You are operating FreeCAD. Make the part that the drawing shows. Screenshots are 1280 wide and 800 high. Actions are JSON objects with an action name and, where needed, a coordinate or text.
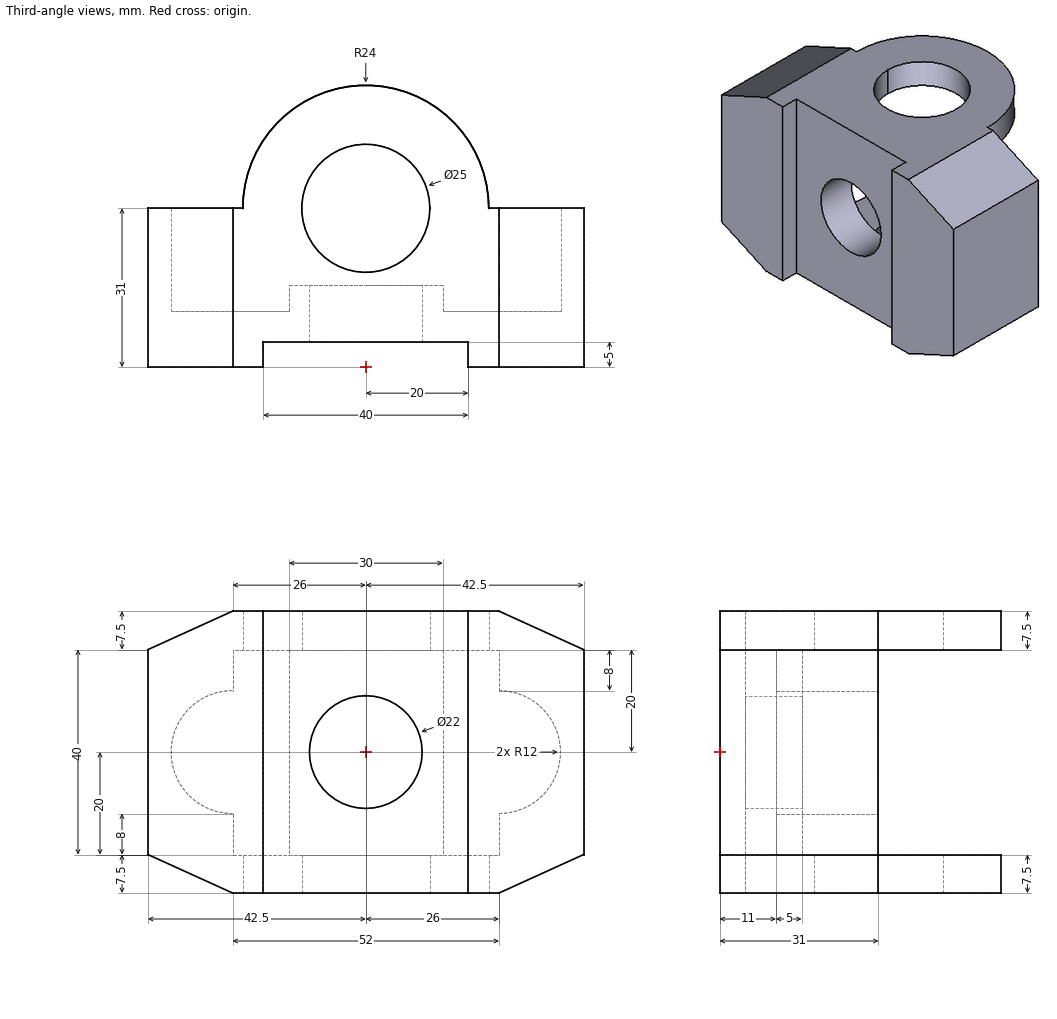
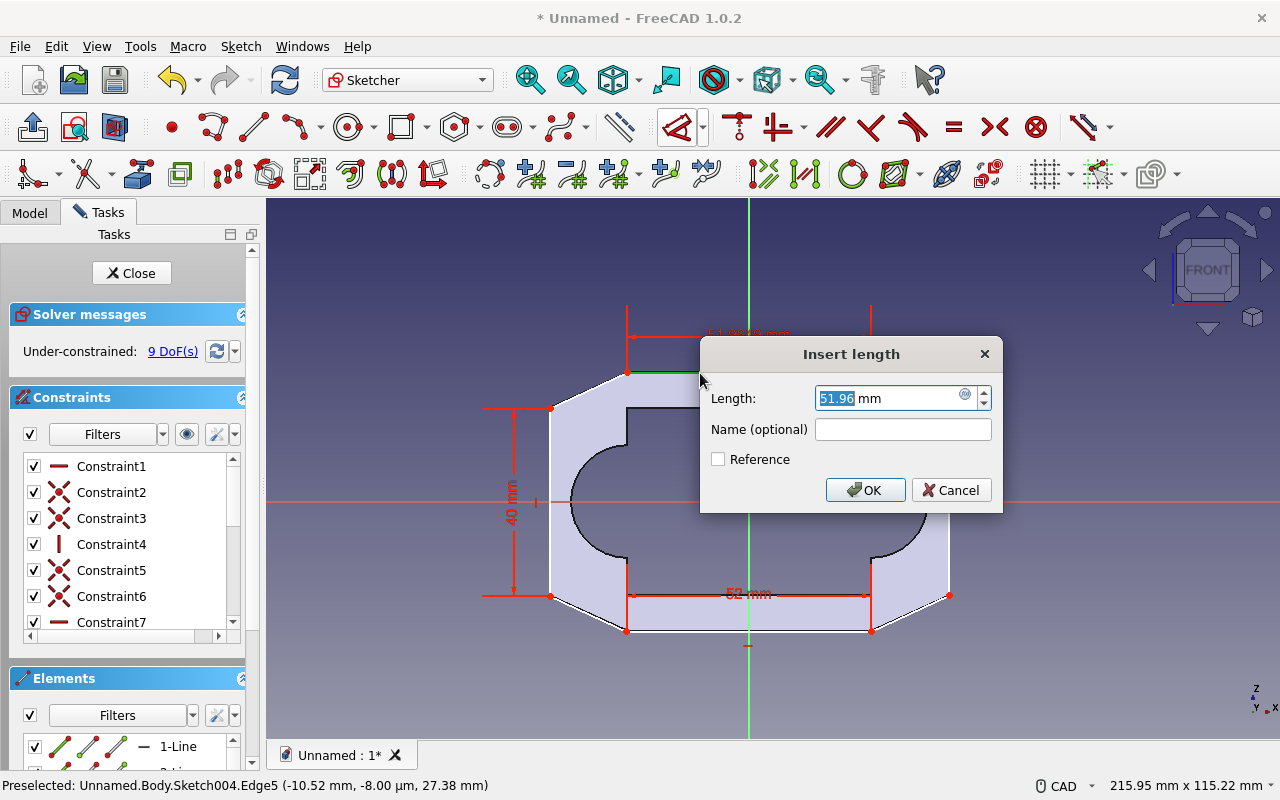
{"action": "type", "text": "52"}
{"action": "key", "text": "Return"}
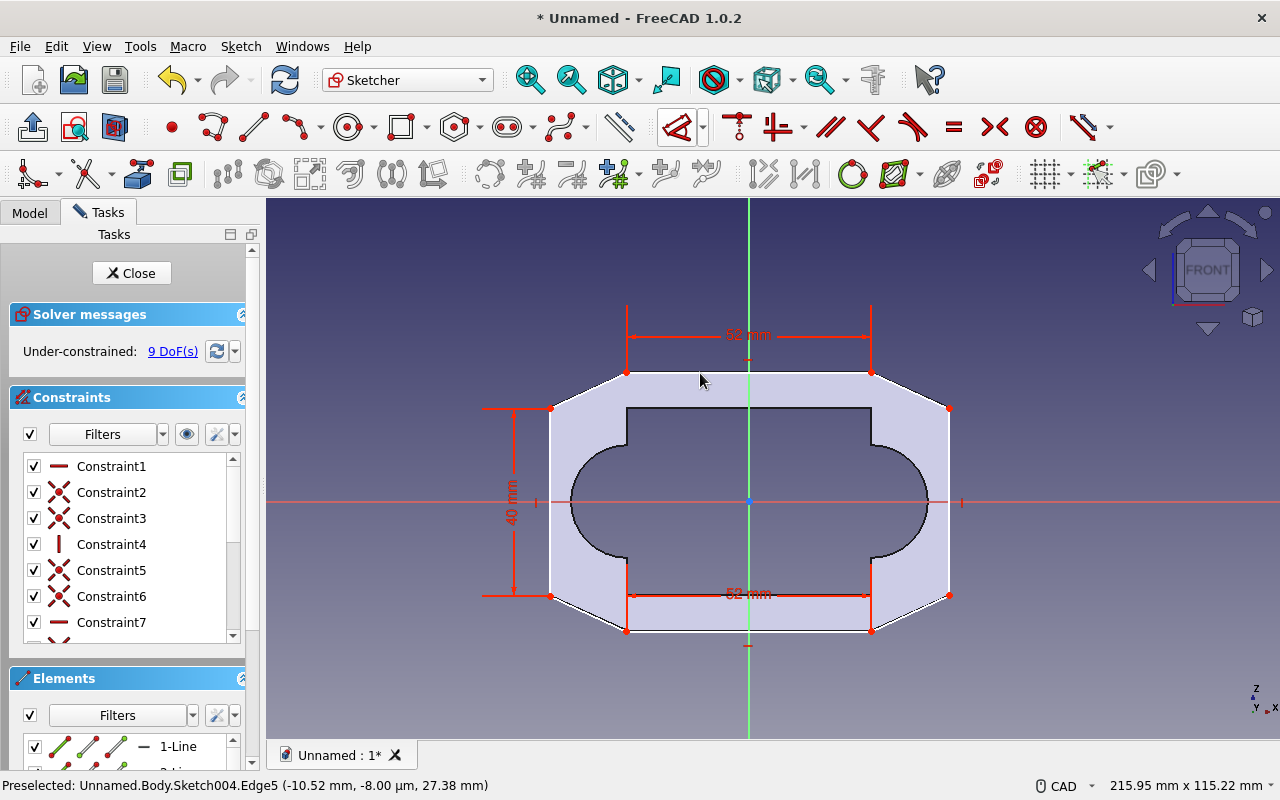
{"action": "left_click", "coordinate": [949, 465]}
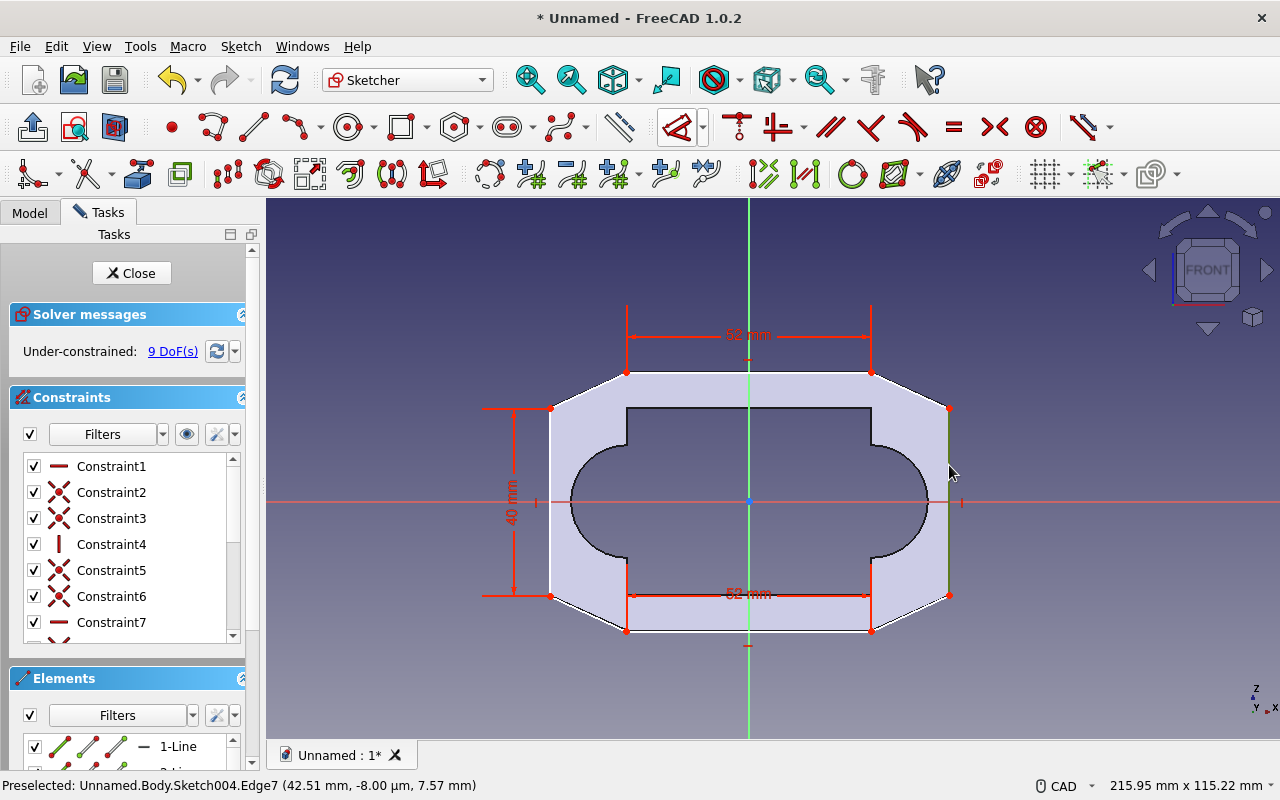
{"action": "key", "text": "i"}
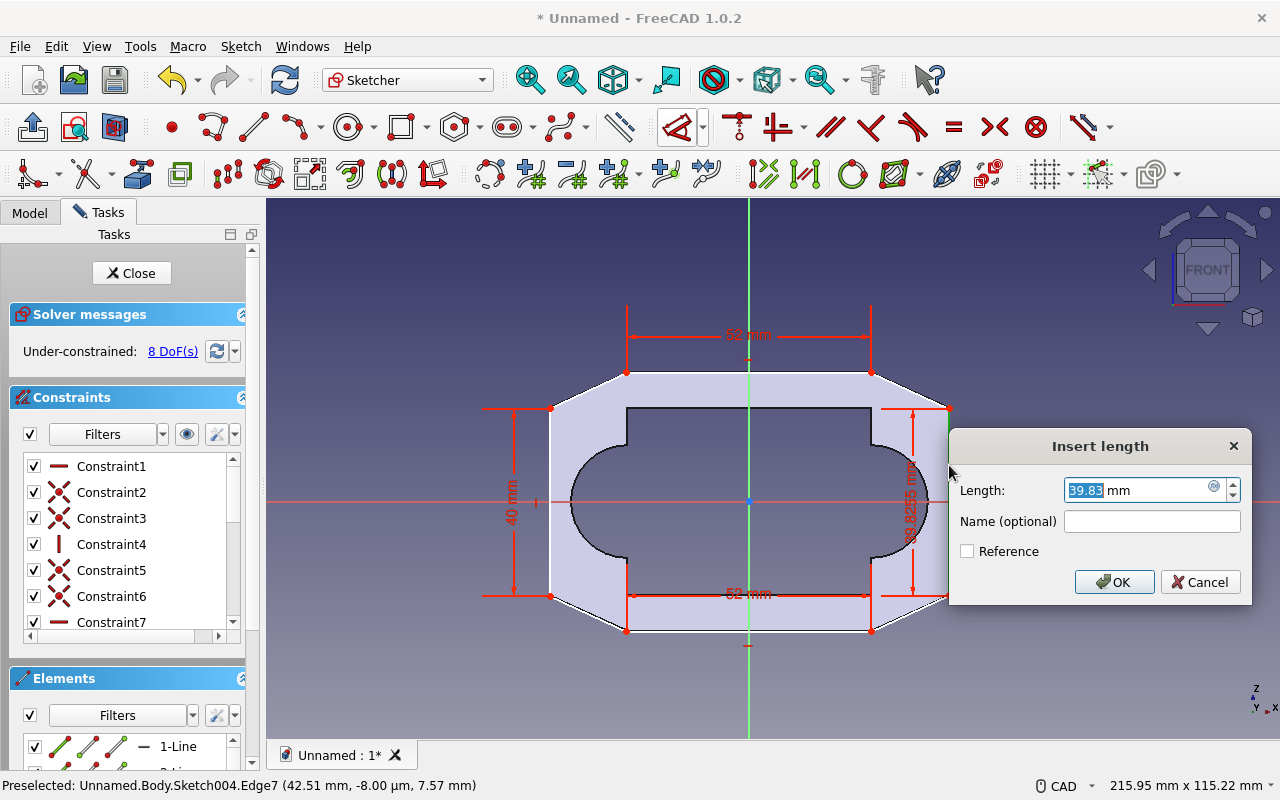
{"action": "type", "text": "40"}
{"action": "key", "text": "Return"}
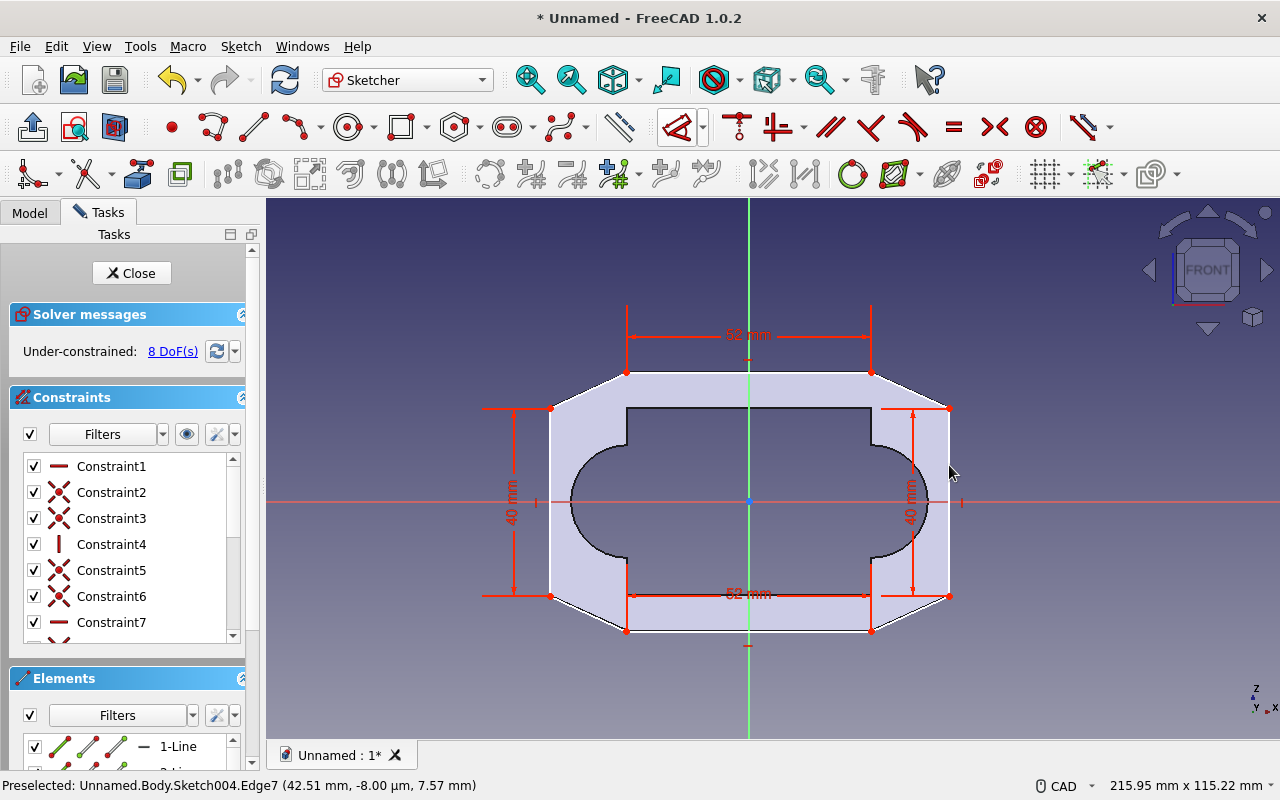
{"action": "left_click", "coordinate": [871, 632]}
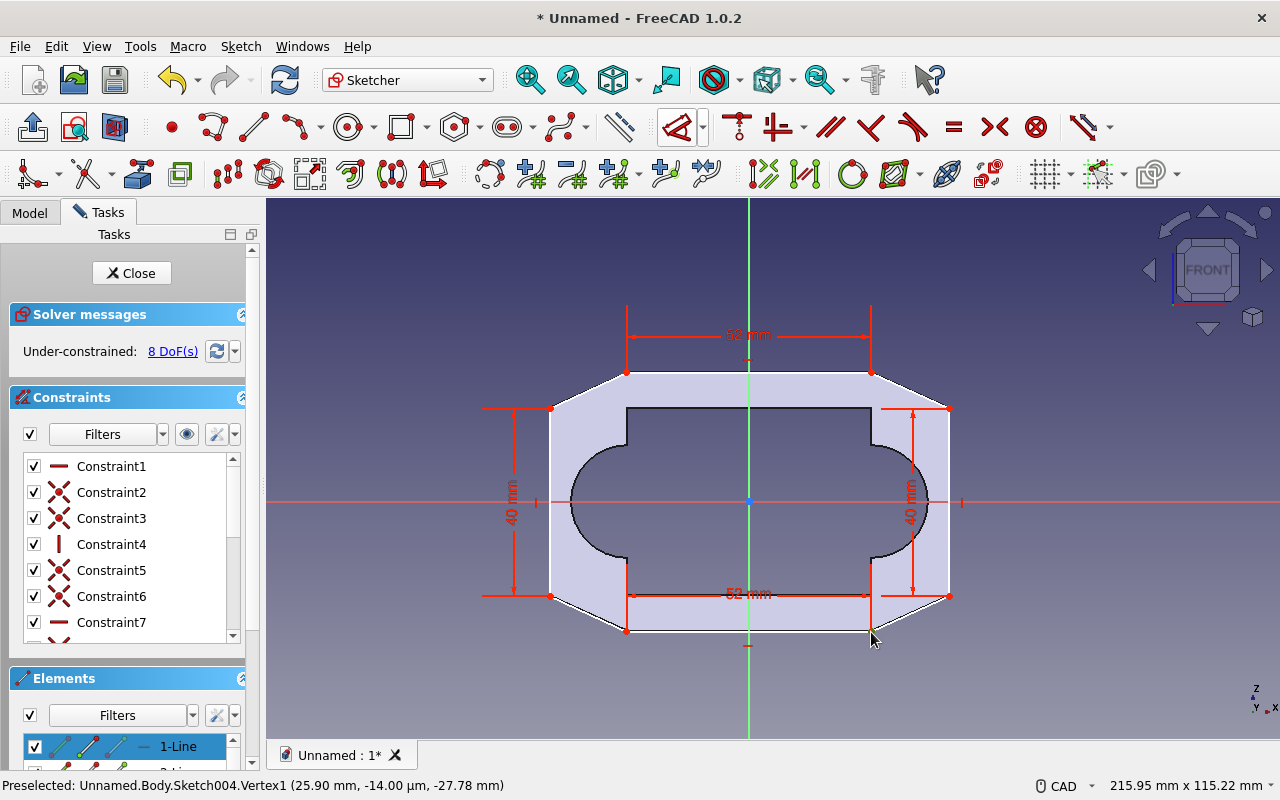
{"action": "key", "text": "l"}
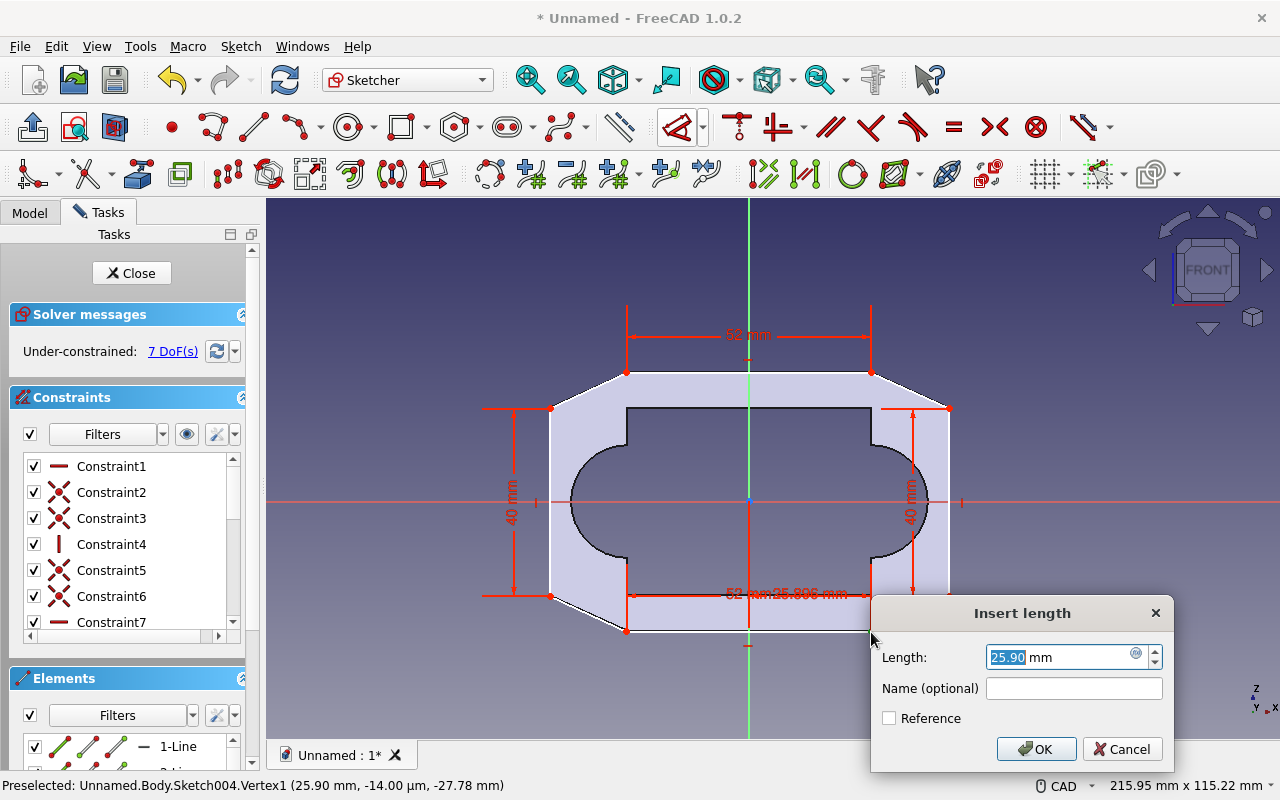
{"action": "type", "text": "26"}
{"action": "key", "text": "Return"}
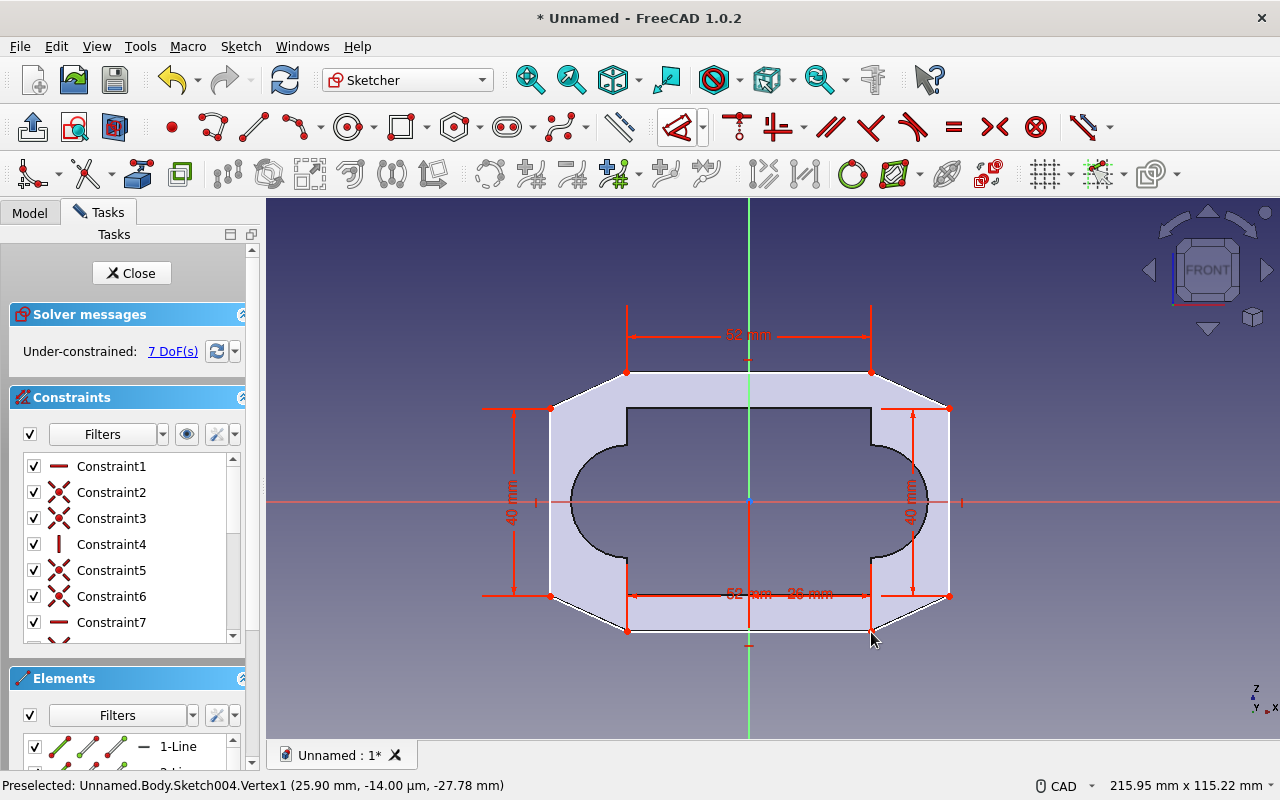
{"action": "left_click", "coordinate": [550, 596]}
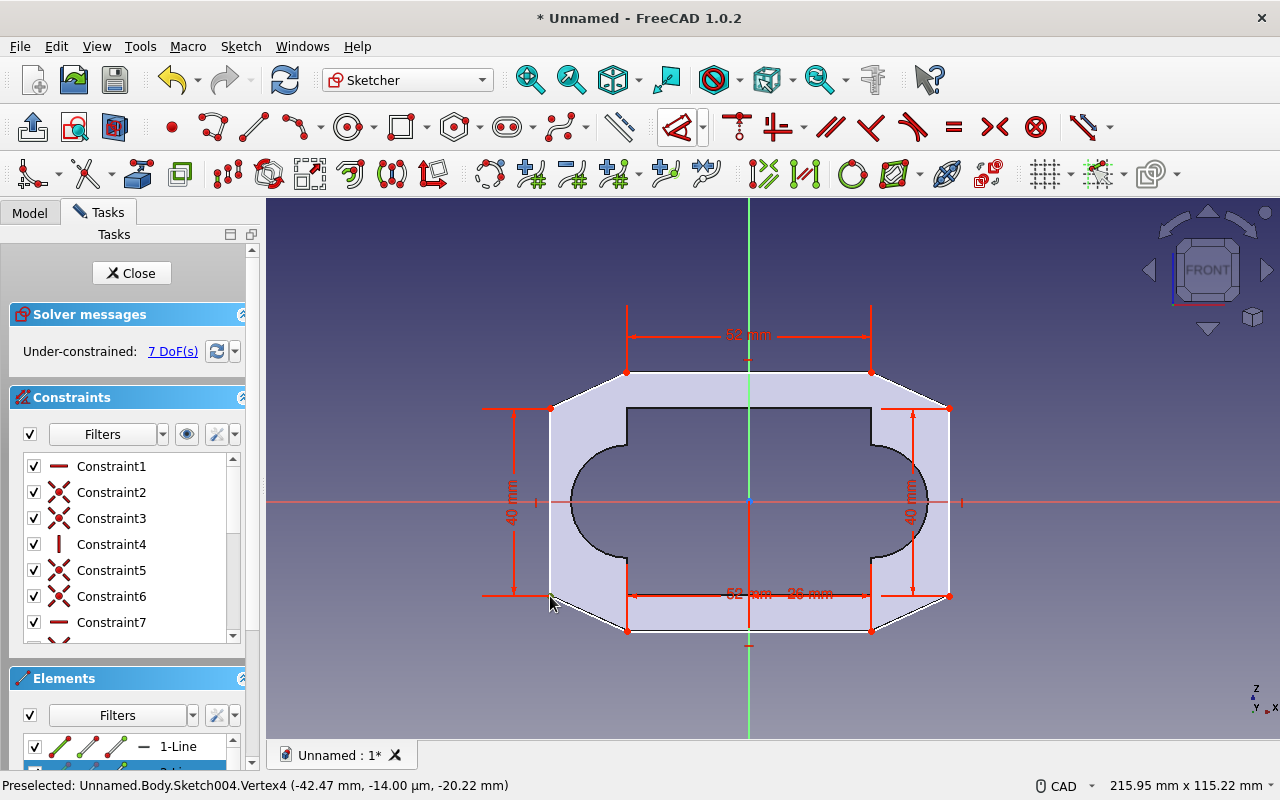
{"action": "key", "text": "i"}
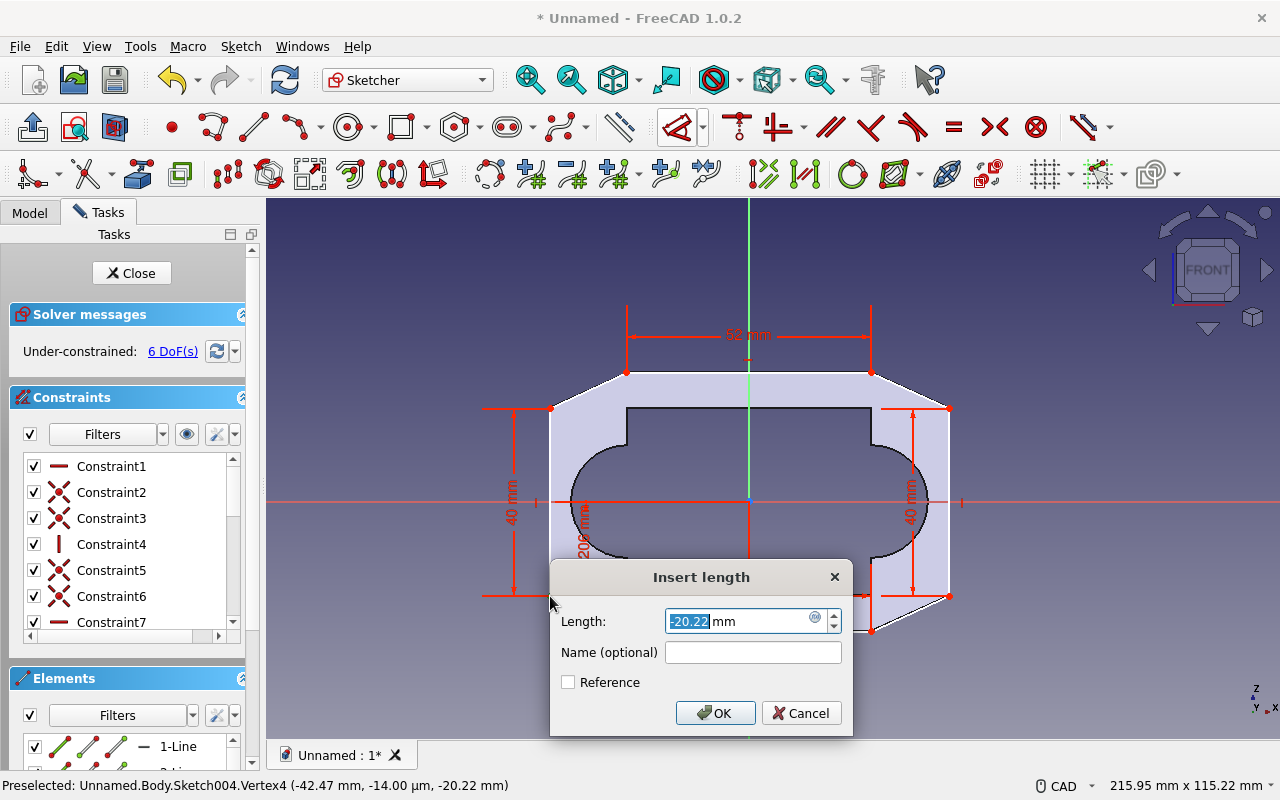
{"action": "type", "text": "-20"}
{"action": "key", "text": "Return"}